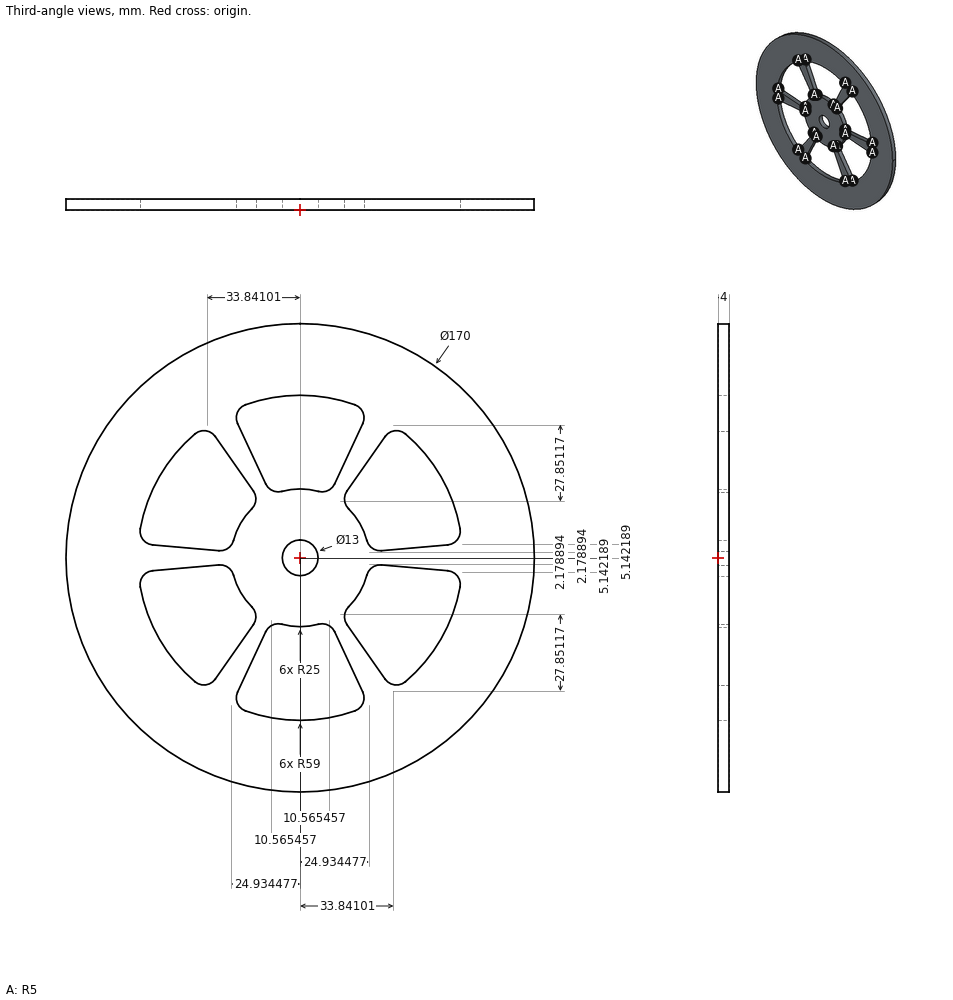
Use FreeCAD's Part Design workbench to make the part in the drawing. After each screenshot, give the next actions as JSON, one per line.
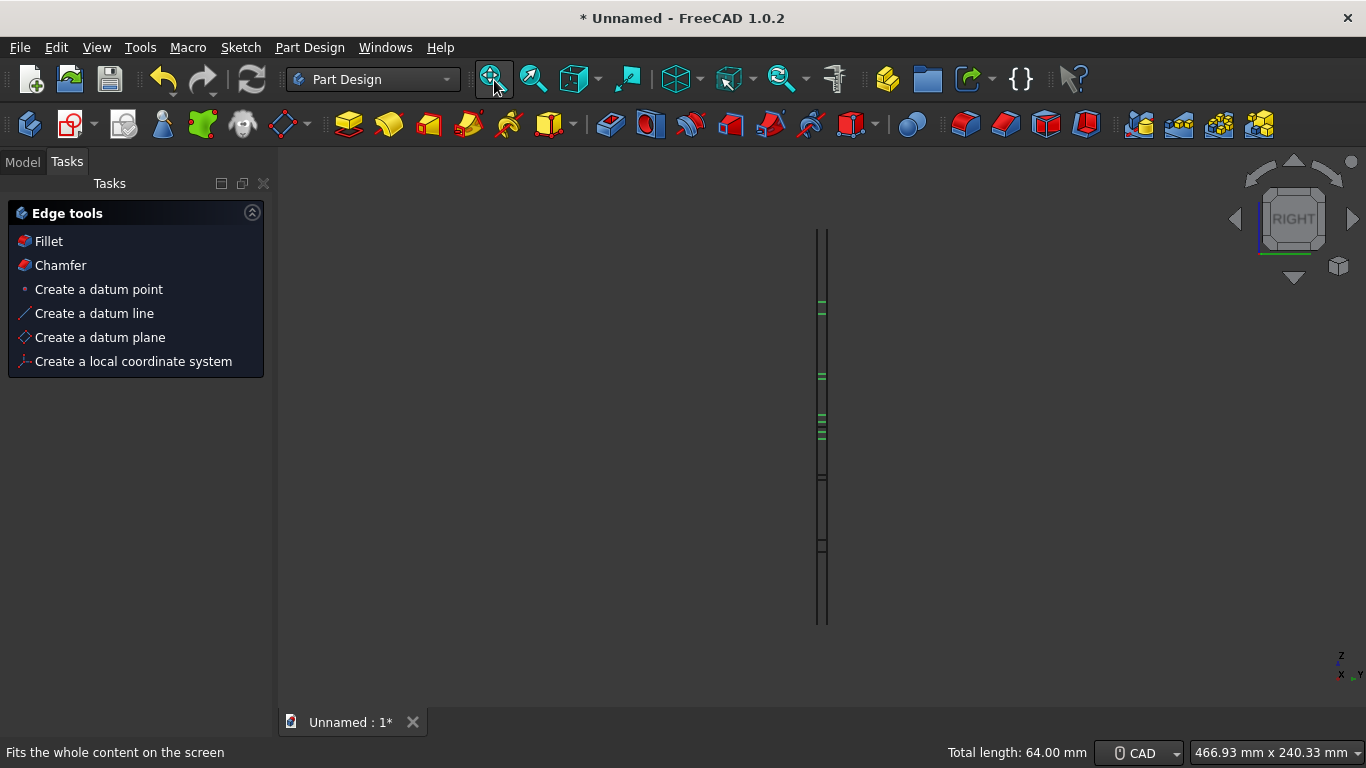
{"action": "key", "text": "5"}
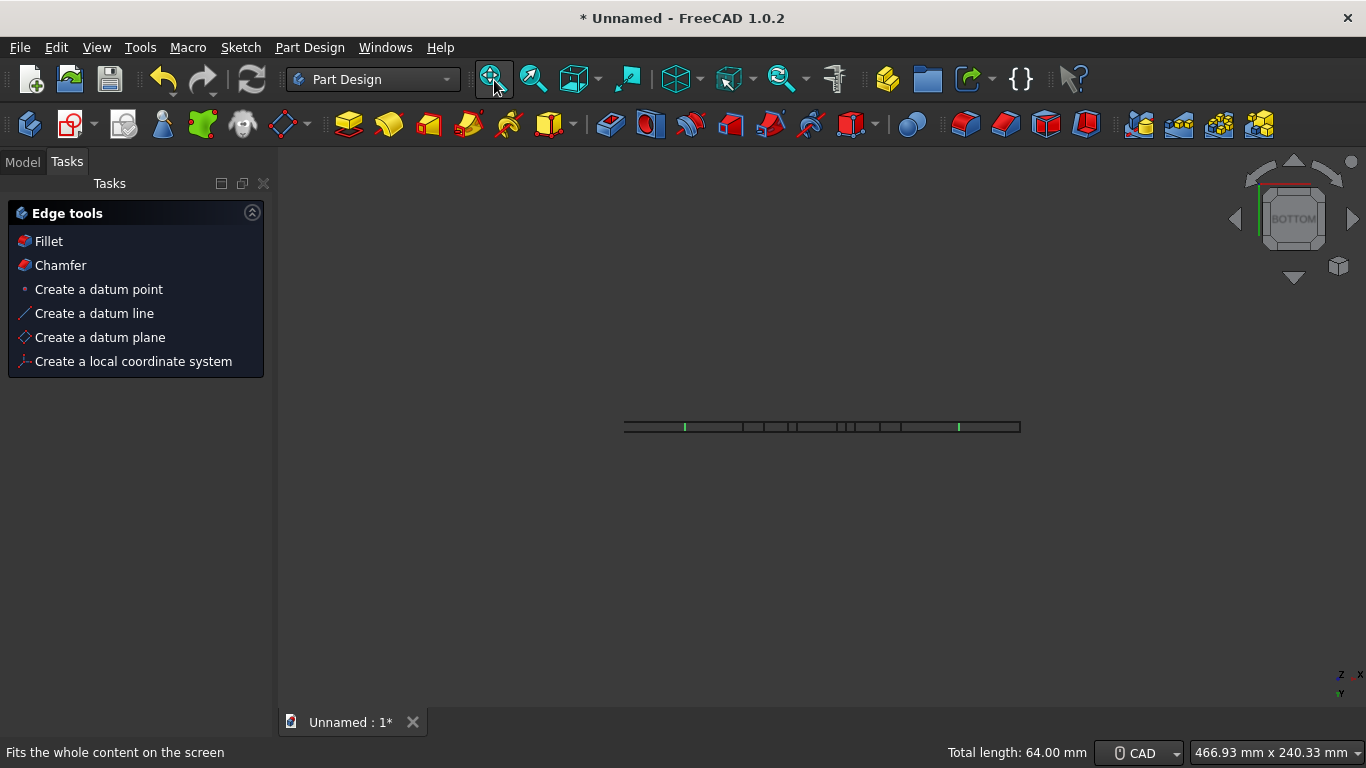
{"action": "left_click", "coordinate": [494, 80]}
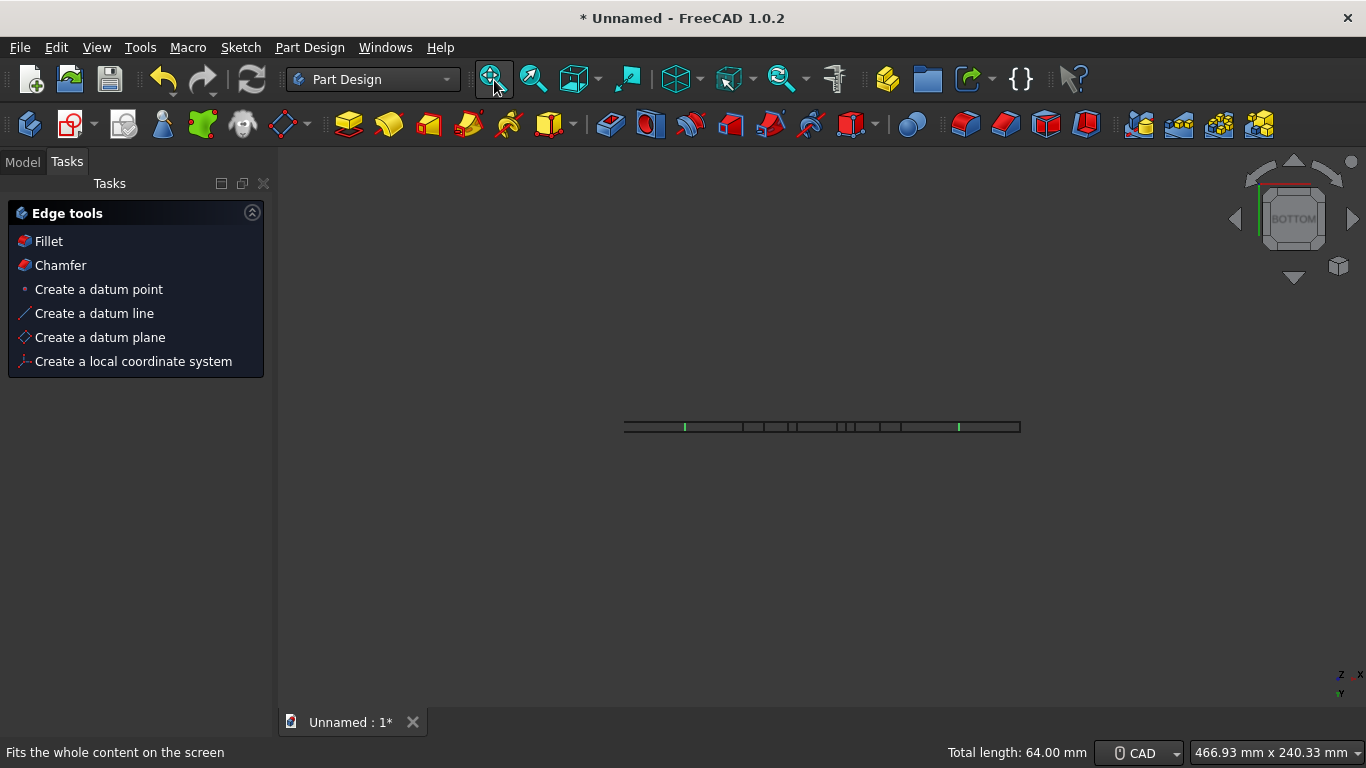
{"action": "scroll", "coordinate": [855, 426], "scroll_direction": "up", "scroll_amount": 8}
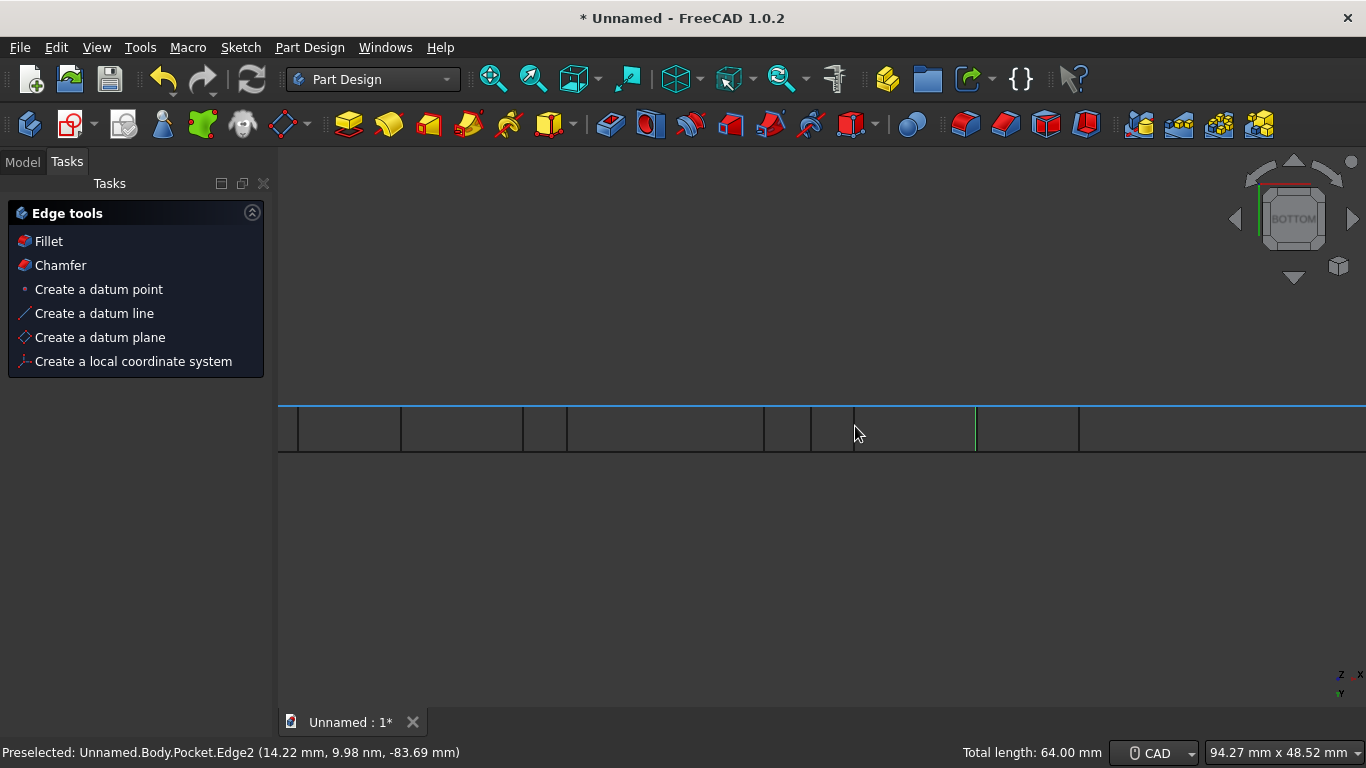
{"action": "left_click", "coordinate": [854, 428], "text": "ctrl"}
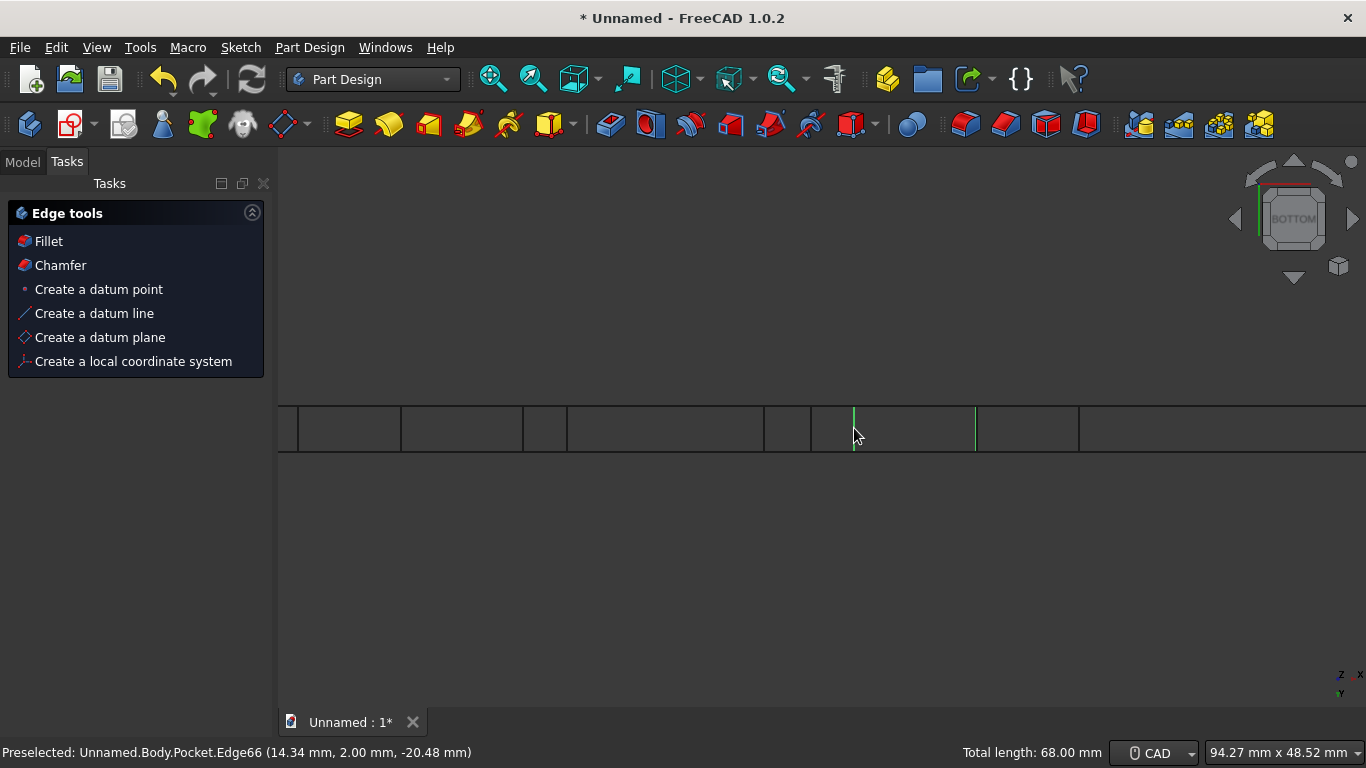
{"action": "left_click", "coordinate": [1079, 428], "text": "ctrl"}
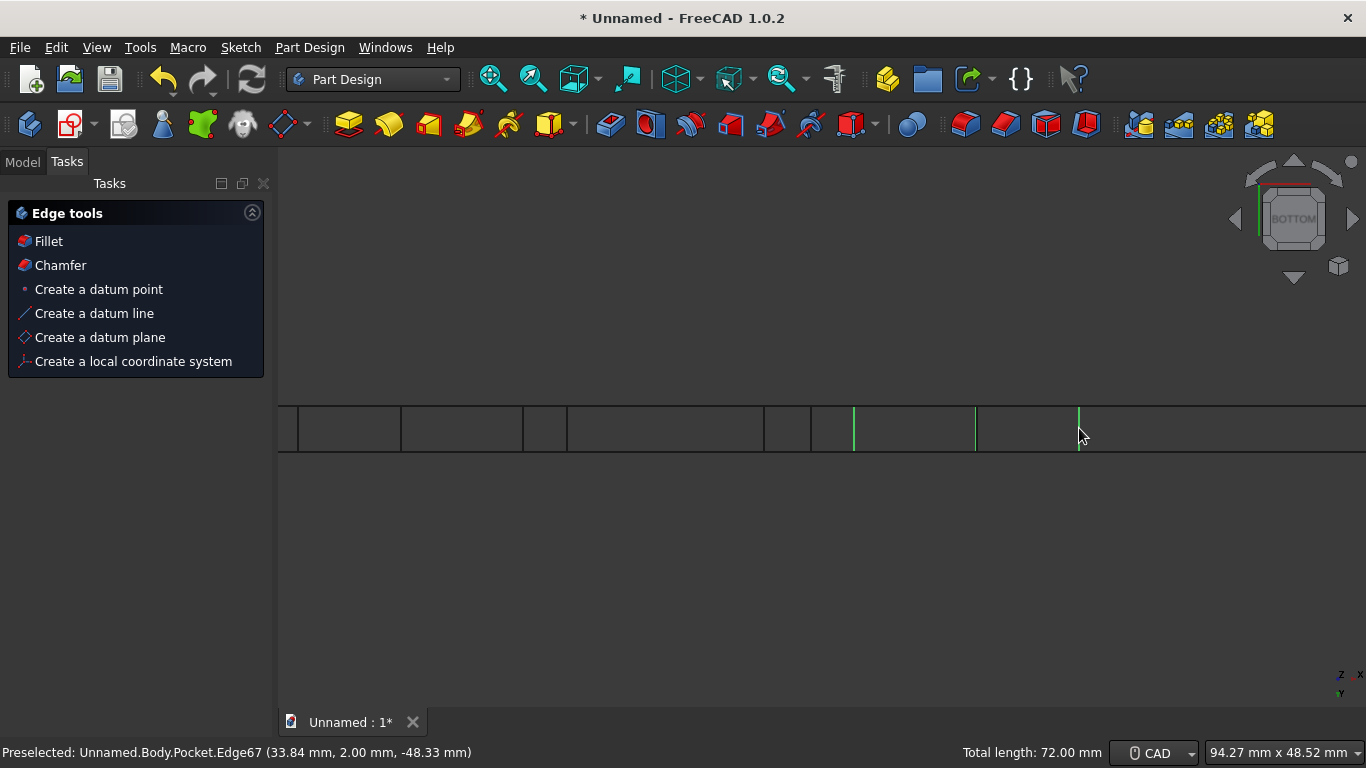
{"action": "left_click", "coordinate": [523, 428], "text": "ctrl"}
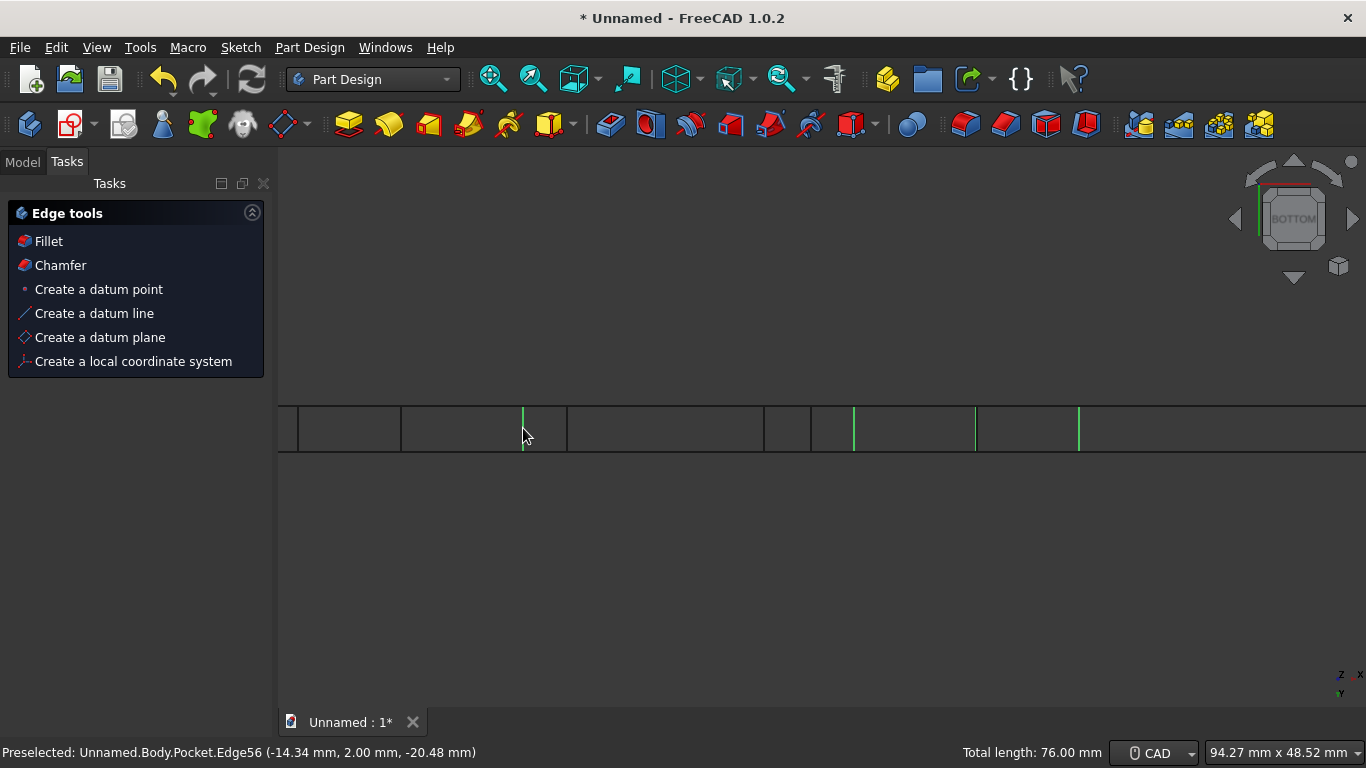
{"action": "left_click", "coordinate": [811, 428], "text": "ctrl"}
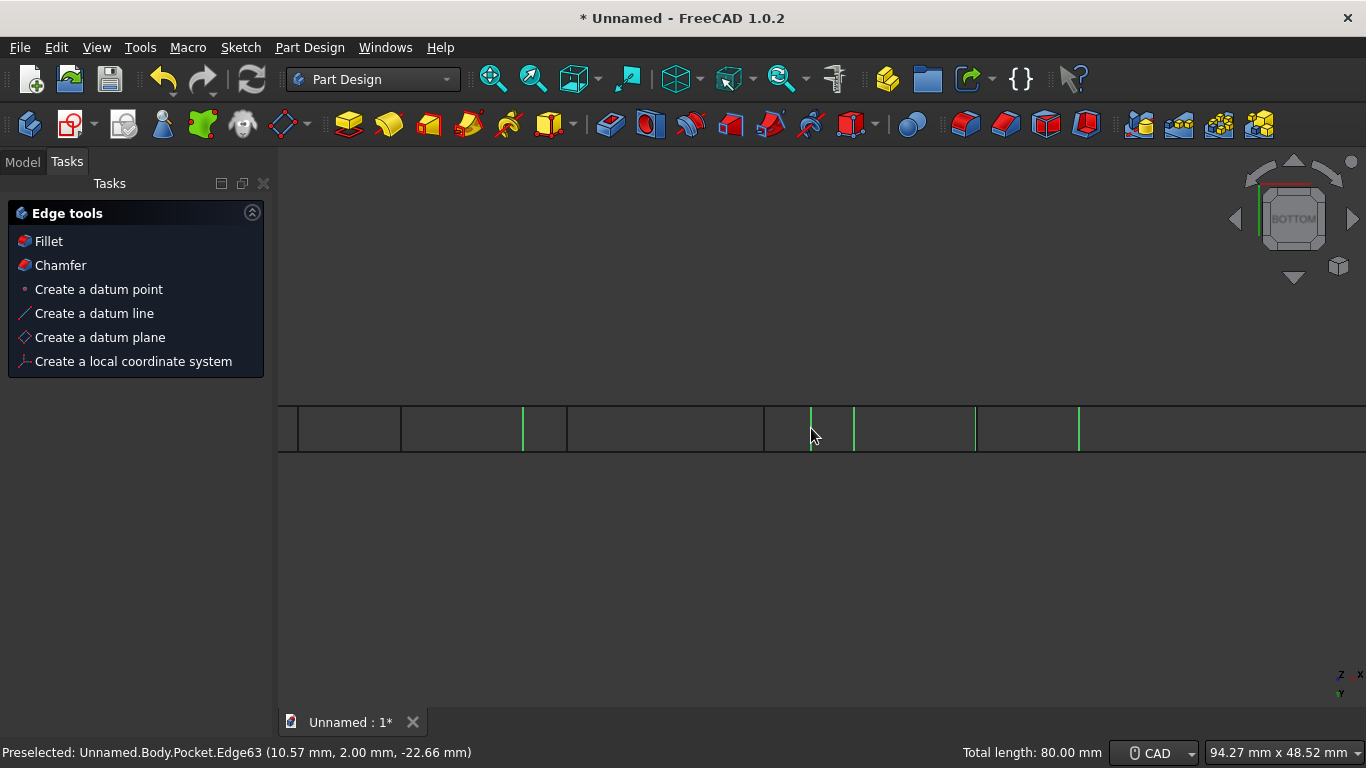
{"action": "left_click", "coordinate": [567, 428], "text": "ctrl"}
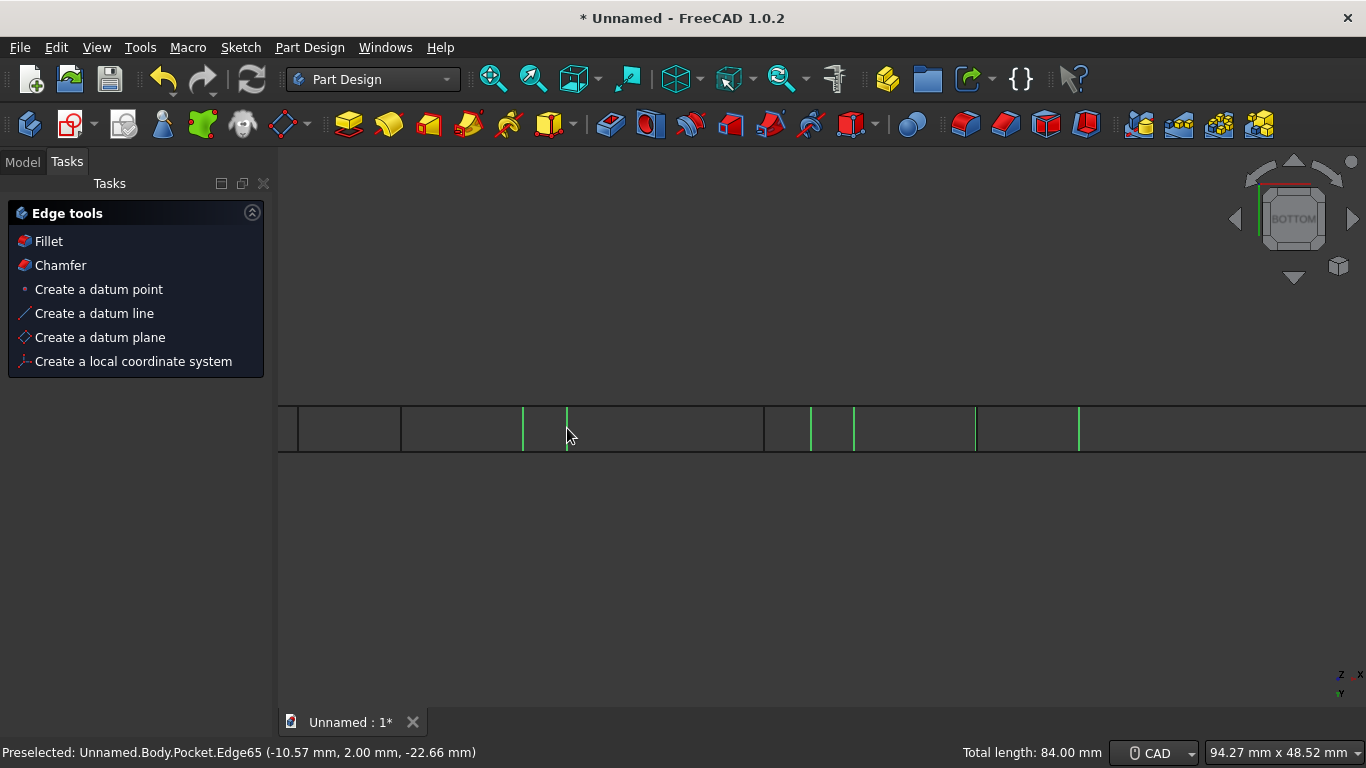
{"action": "left_click", "coordinate": [401, 428], "text": "ctrl"}